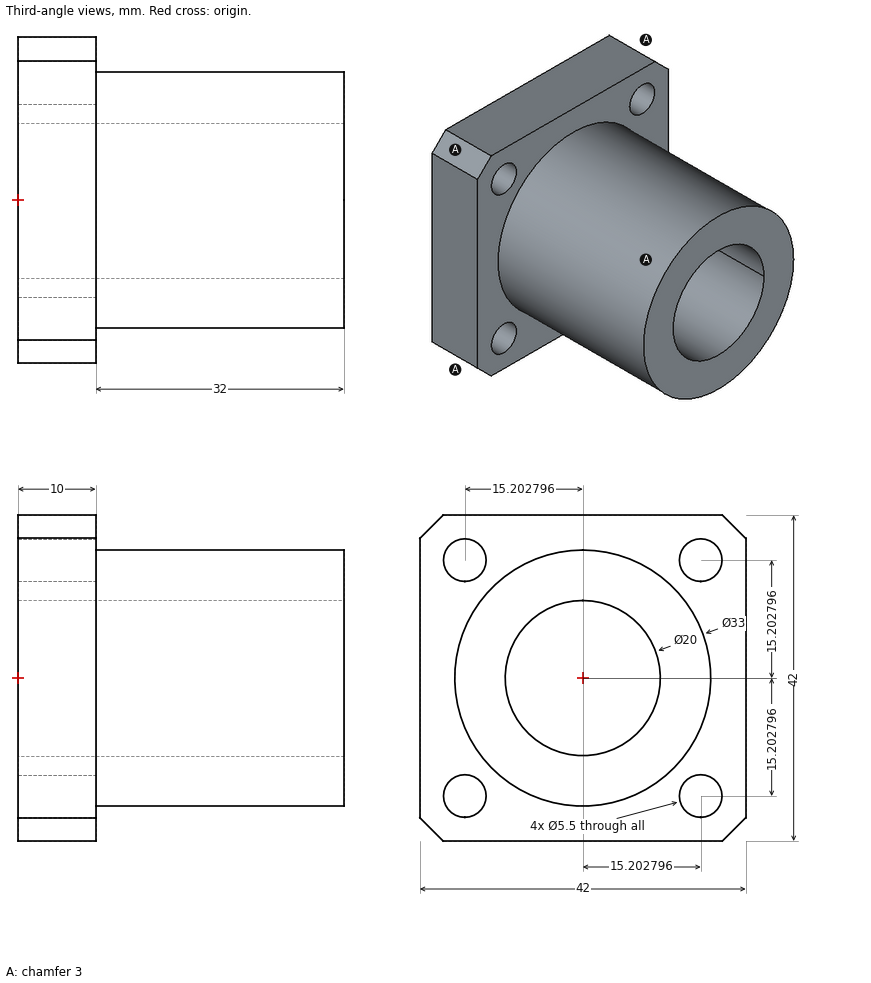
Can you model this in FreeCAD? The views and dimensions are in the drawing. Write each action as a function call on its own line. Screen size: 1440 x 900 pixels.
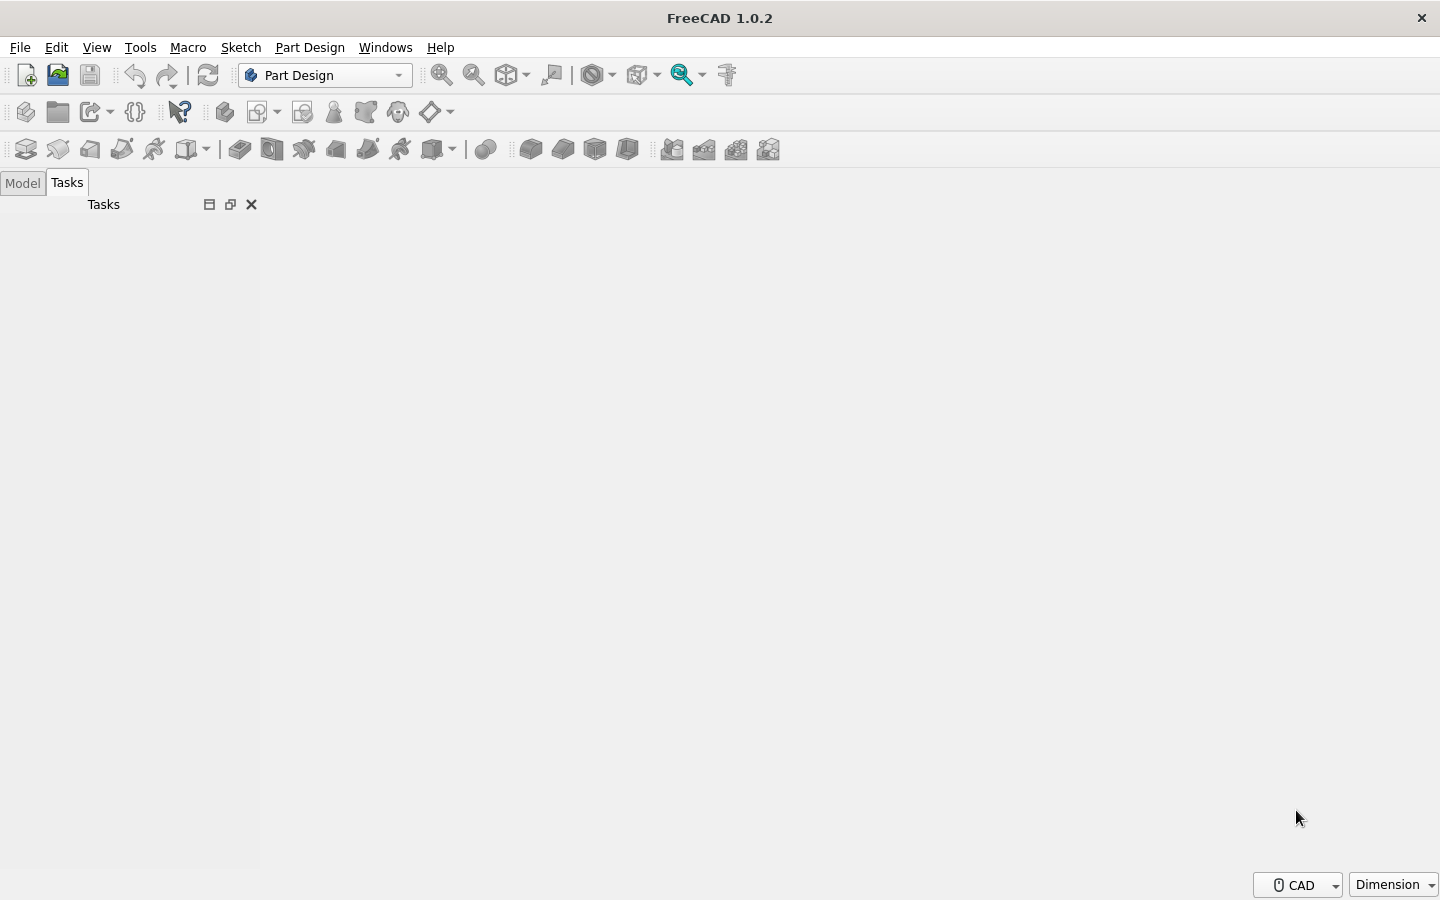
click(26, 76)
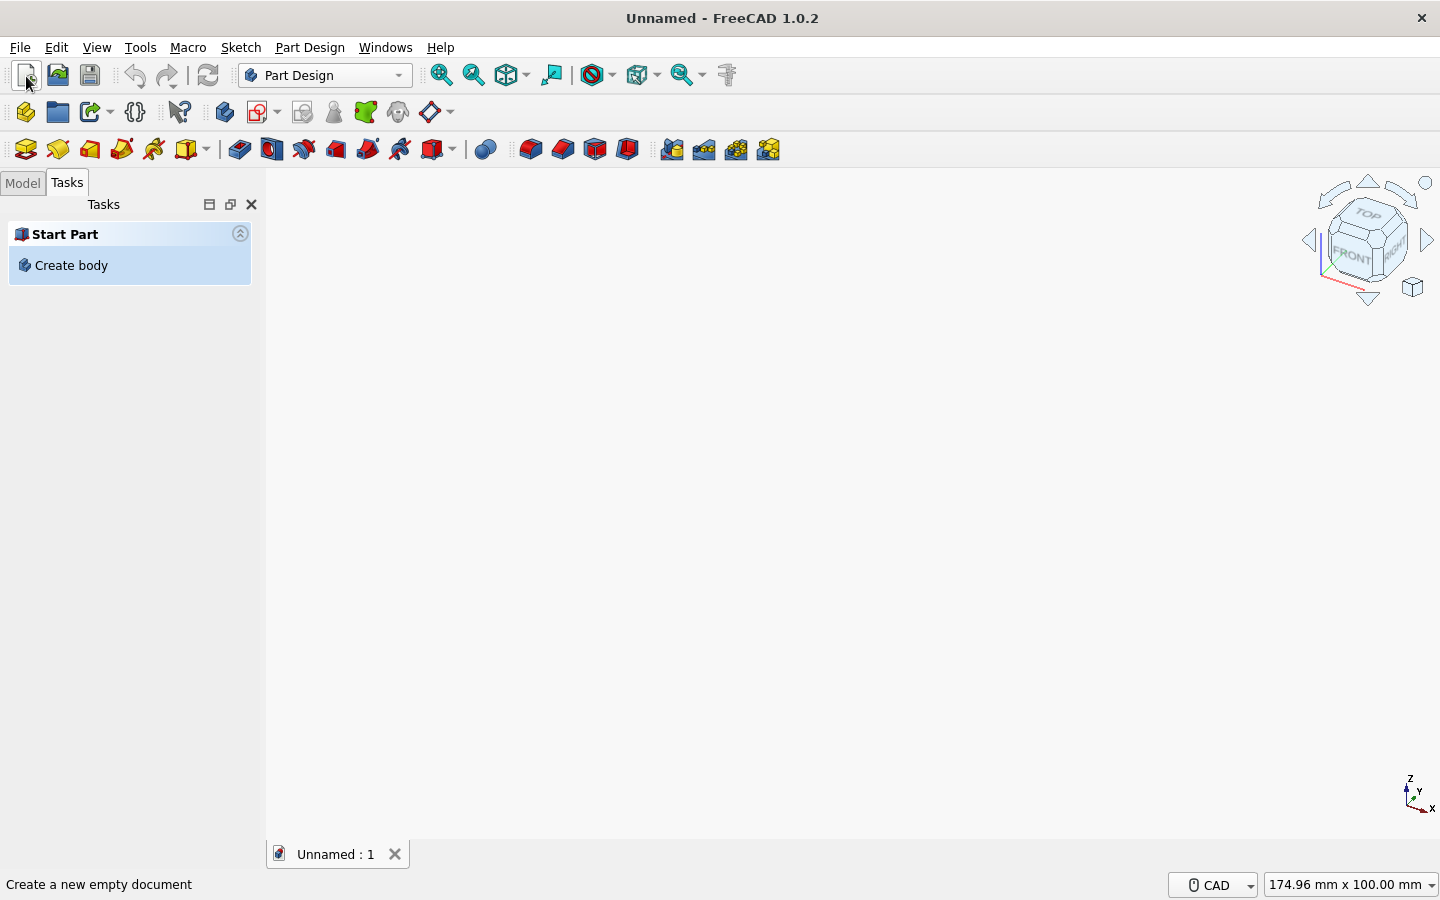
click(258, 112)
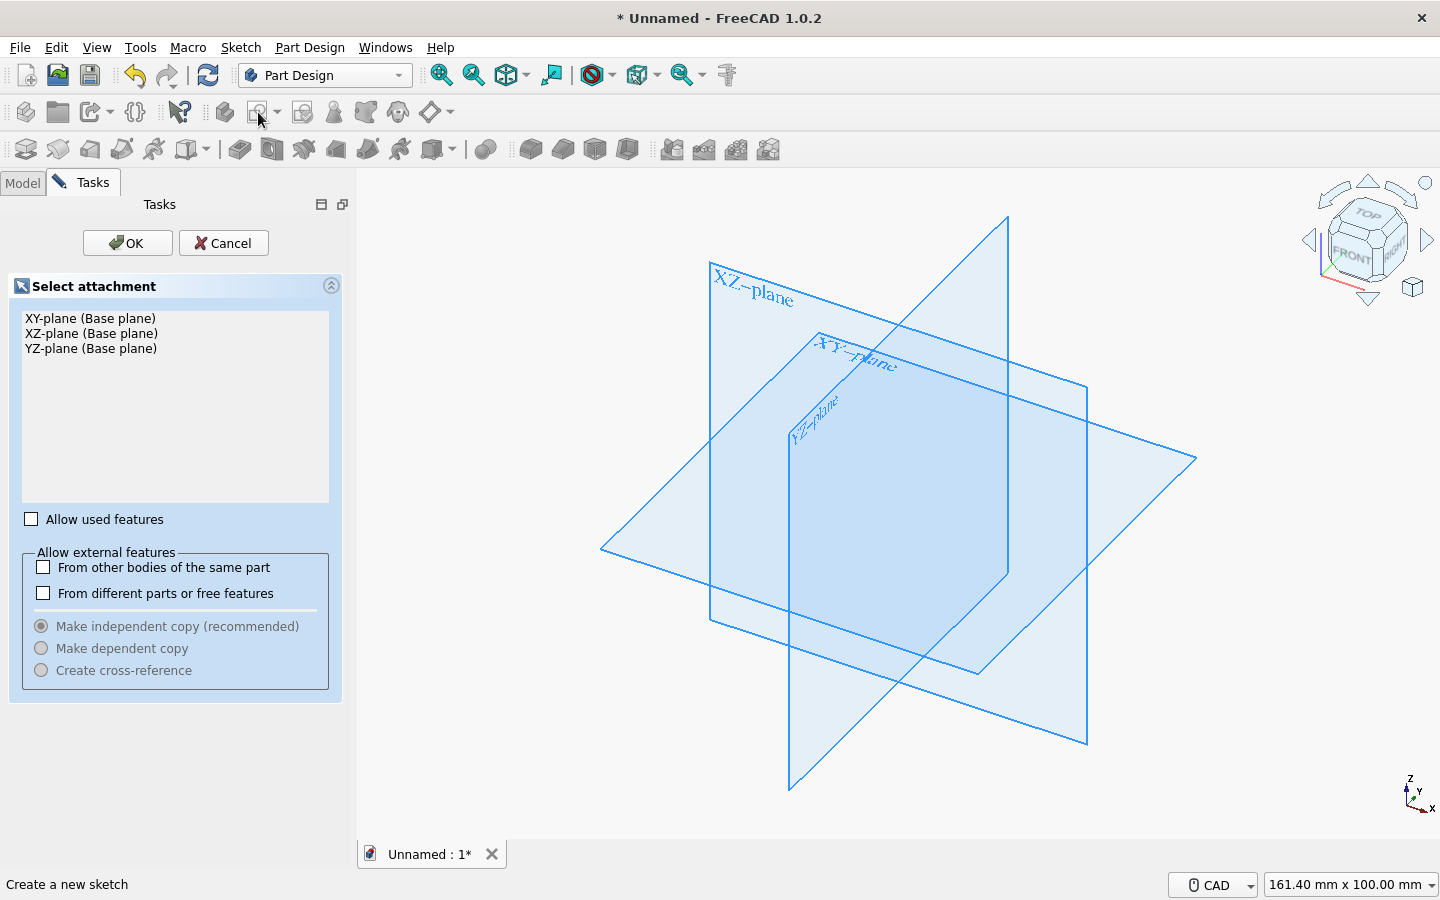
click(82, 348)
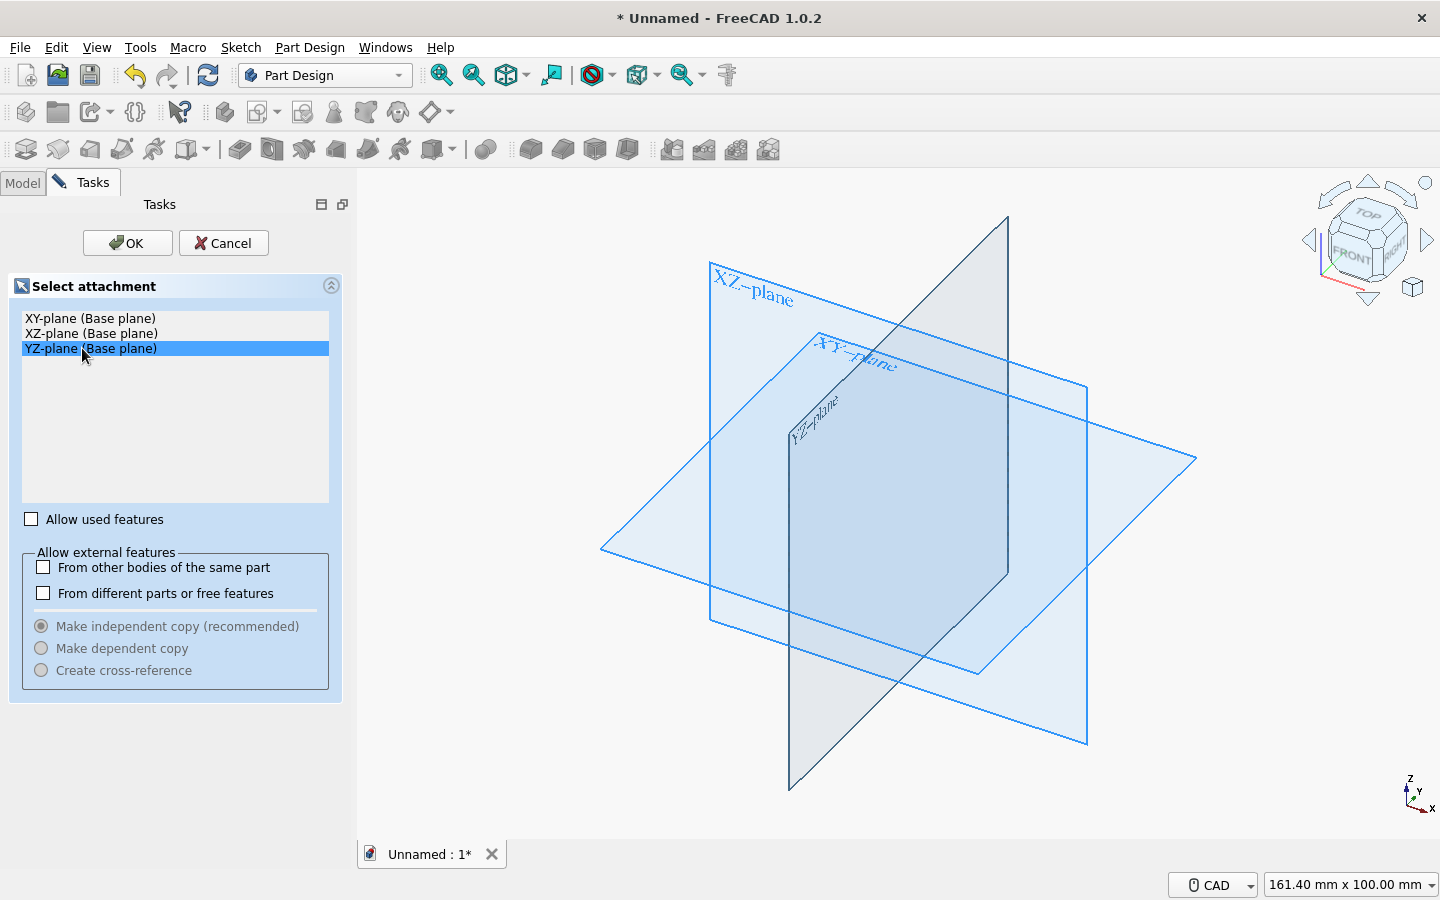
click(128, 243)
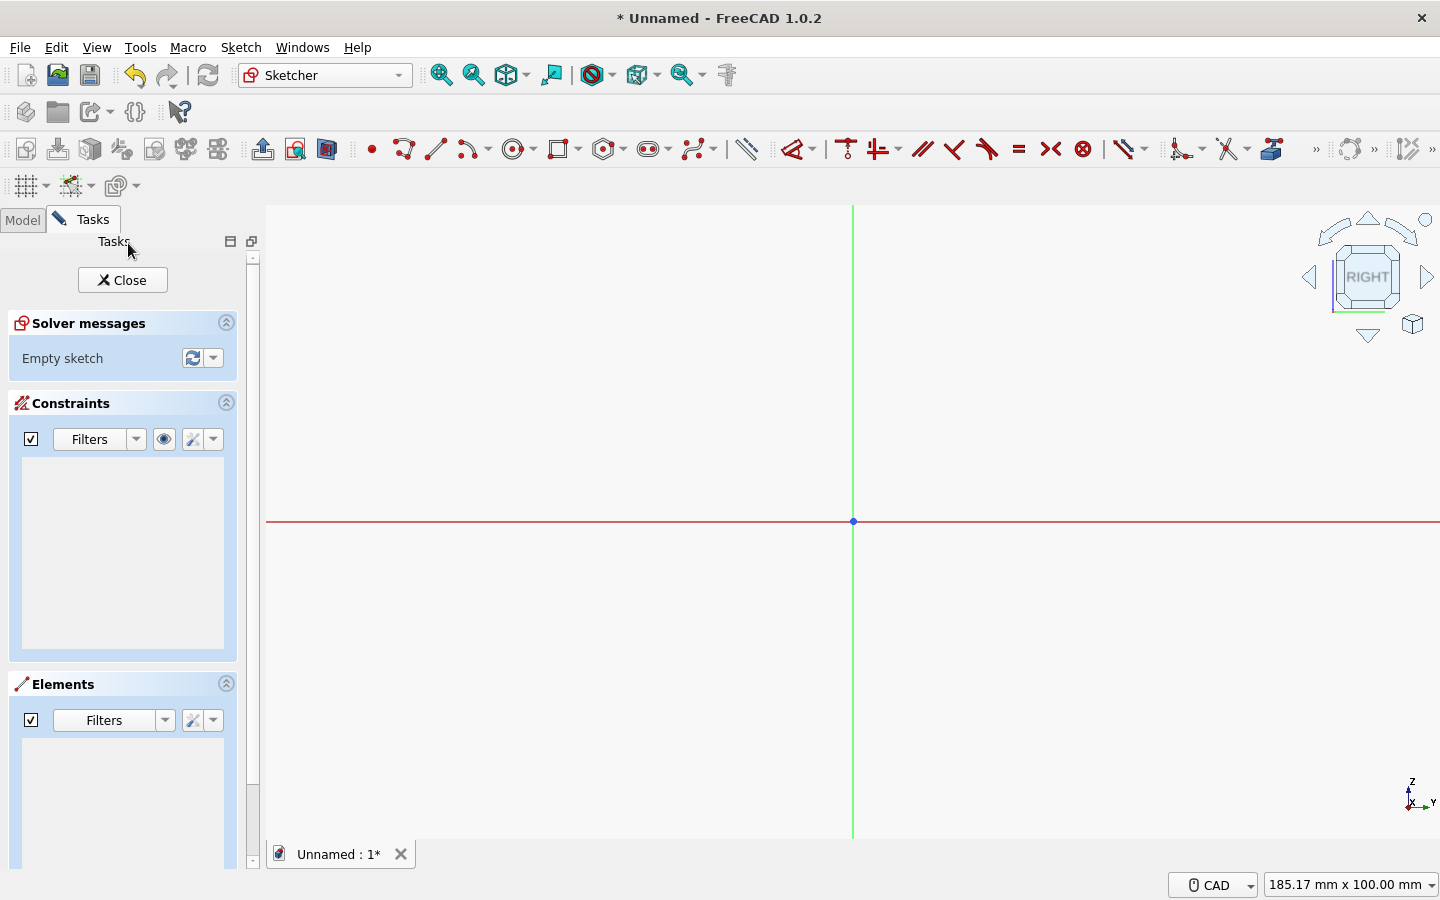
scroll(992, 522, up, 2)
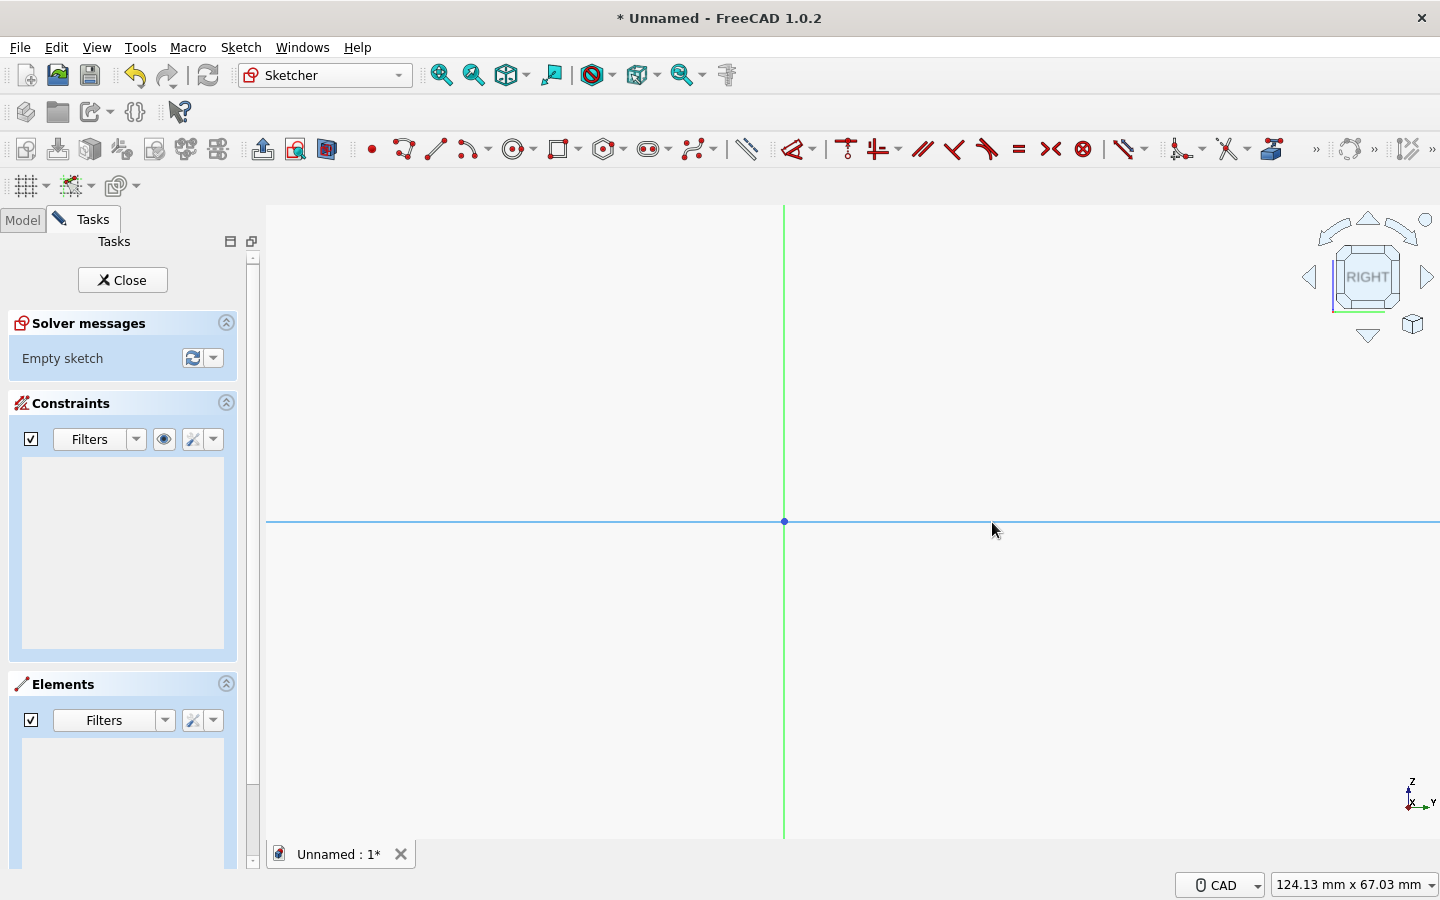
click(580, 150)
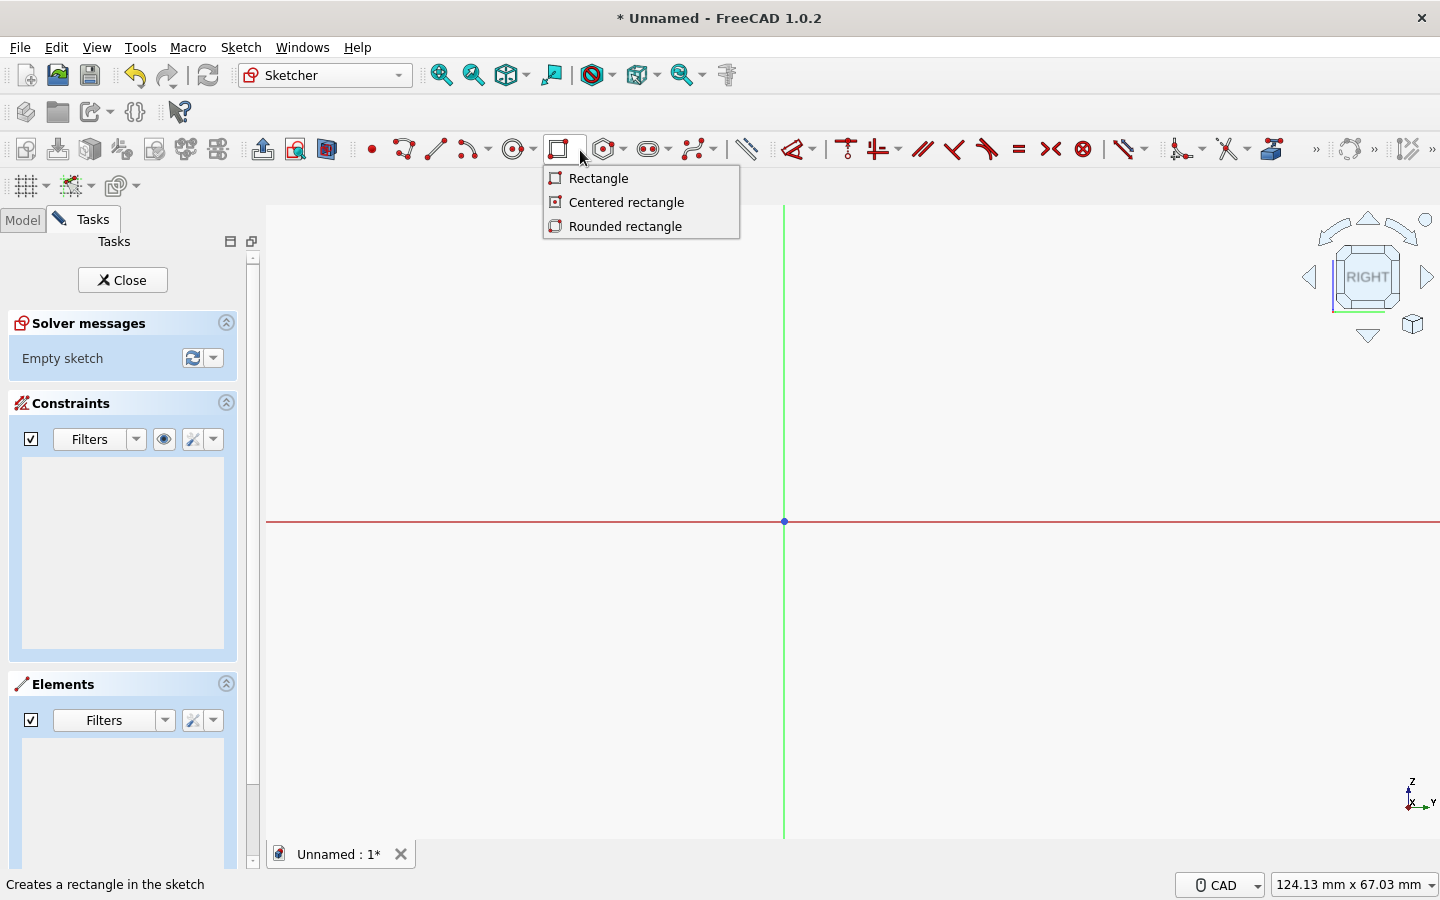
click(642, 202)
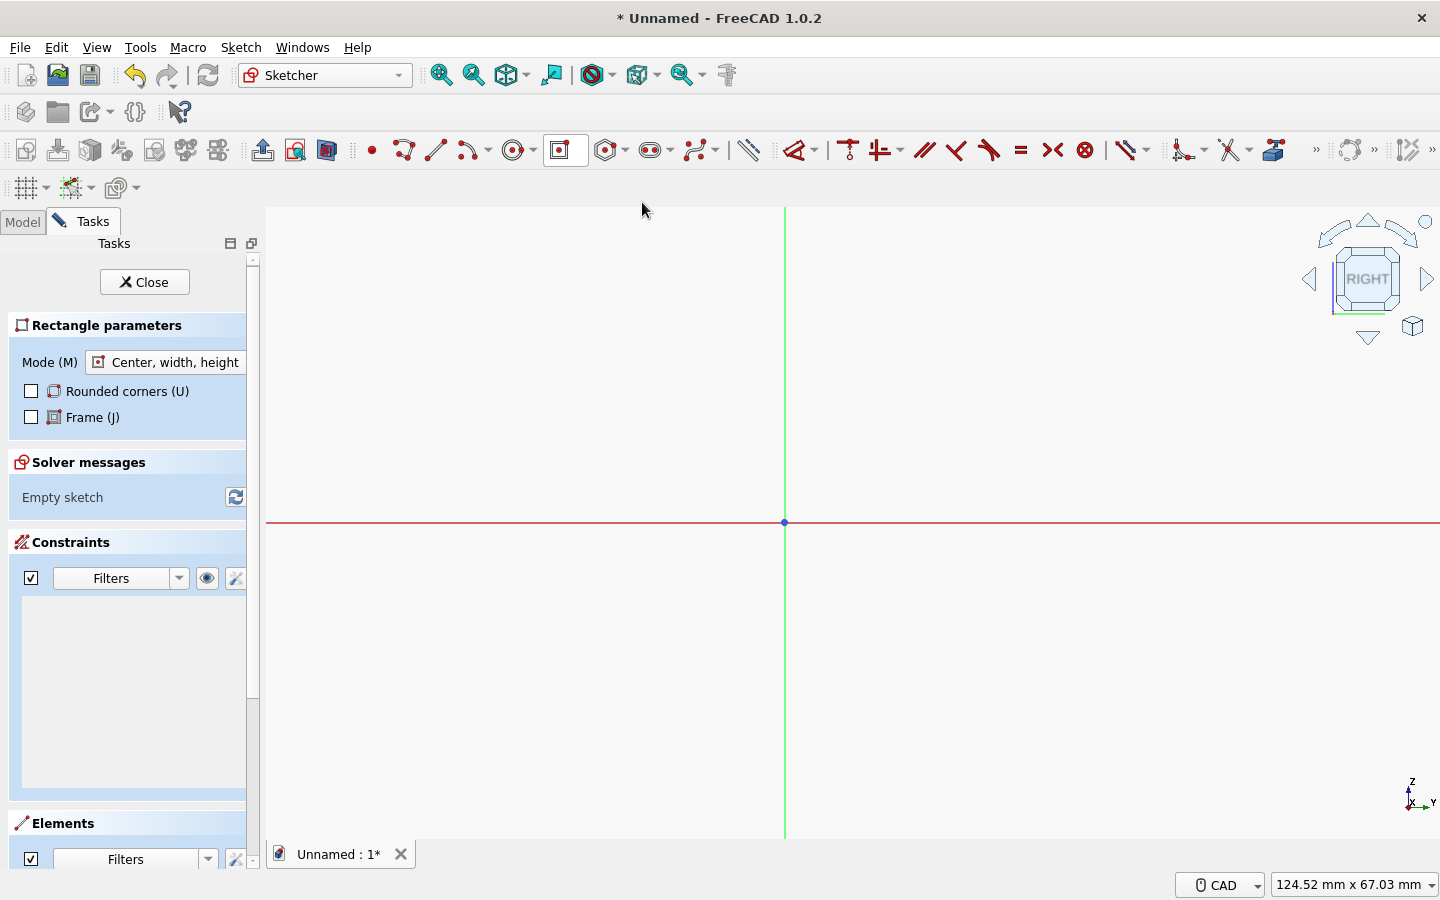
click(785, 523)
click(983, 325)
key(Escape)